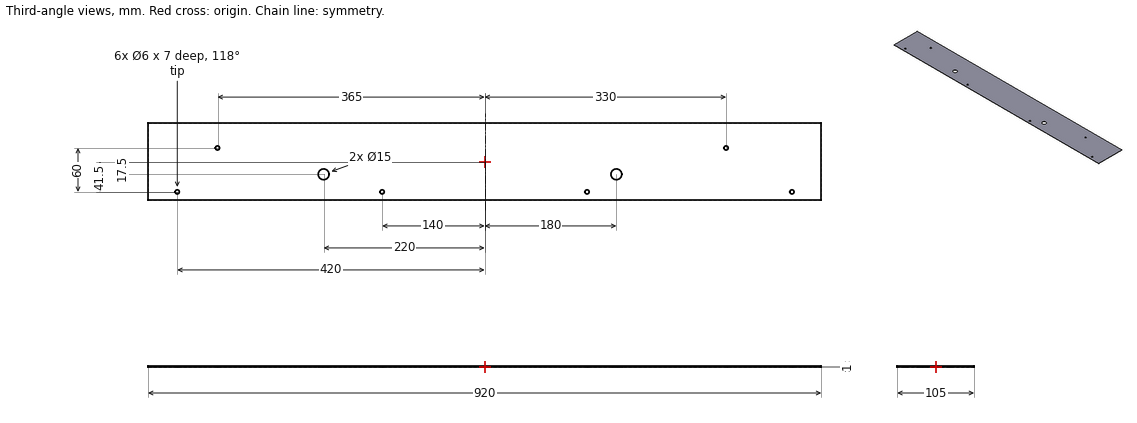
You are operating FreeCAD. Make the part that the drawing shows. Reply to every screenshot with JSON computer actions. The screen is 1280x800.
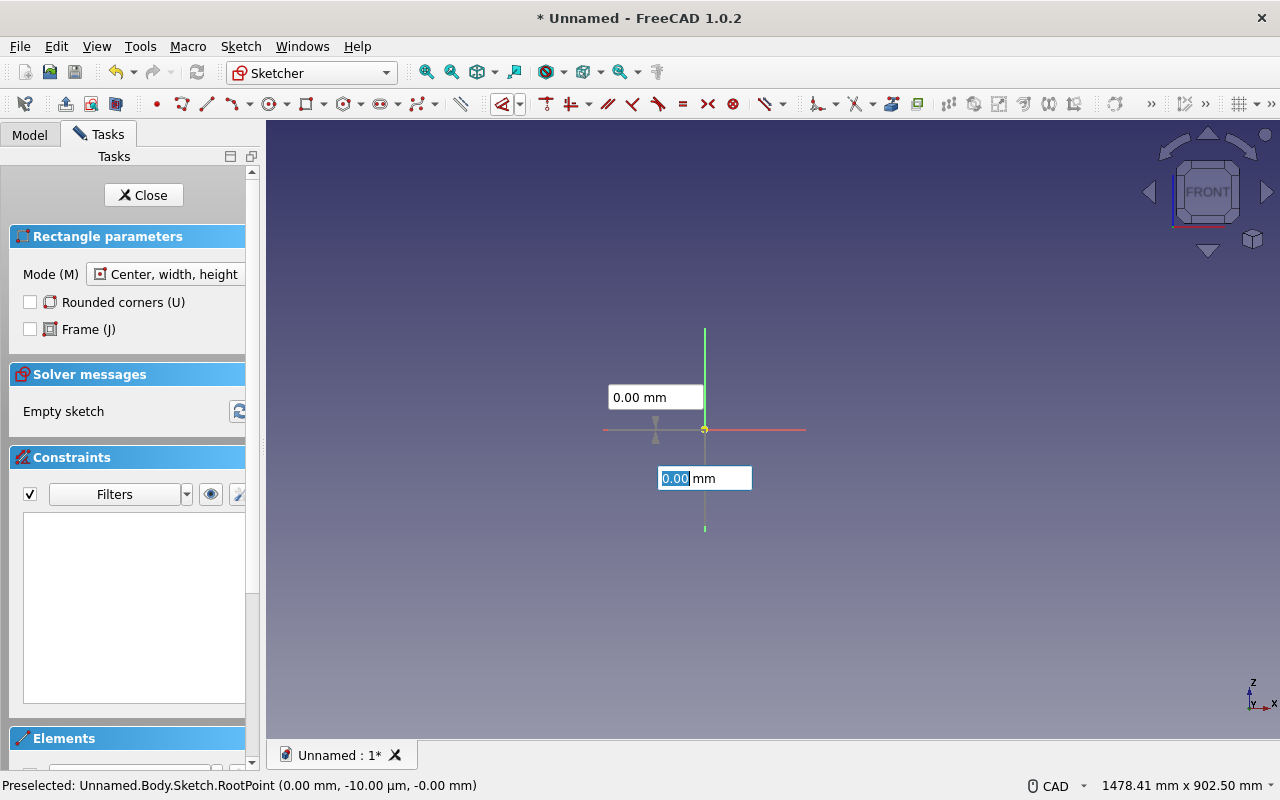
{"action": "scroll", "coordinate": [1020, 429], "scroll_direction": "up", "scroll_amount": 20}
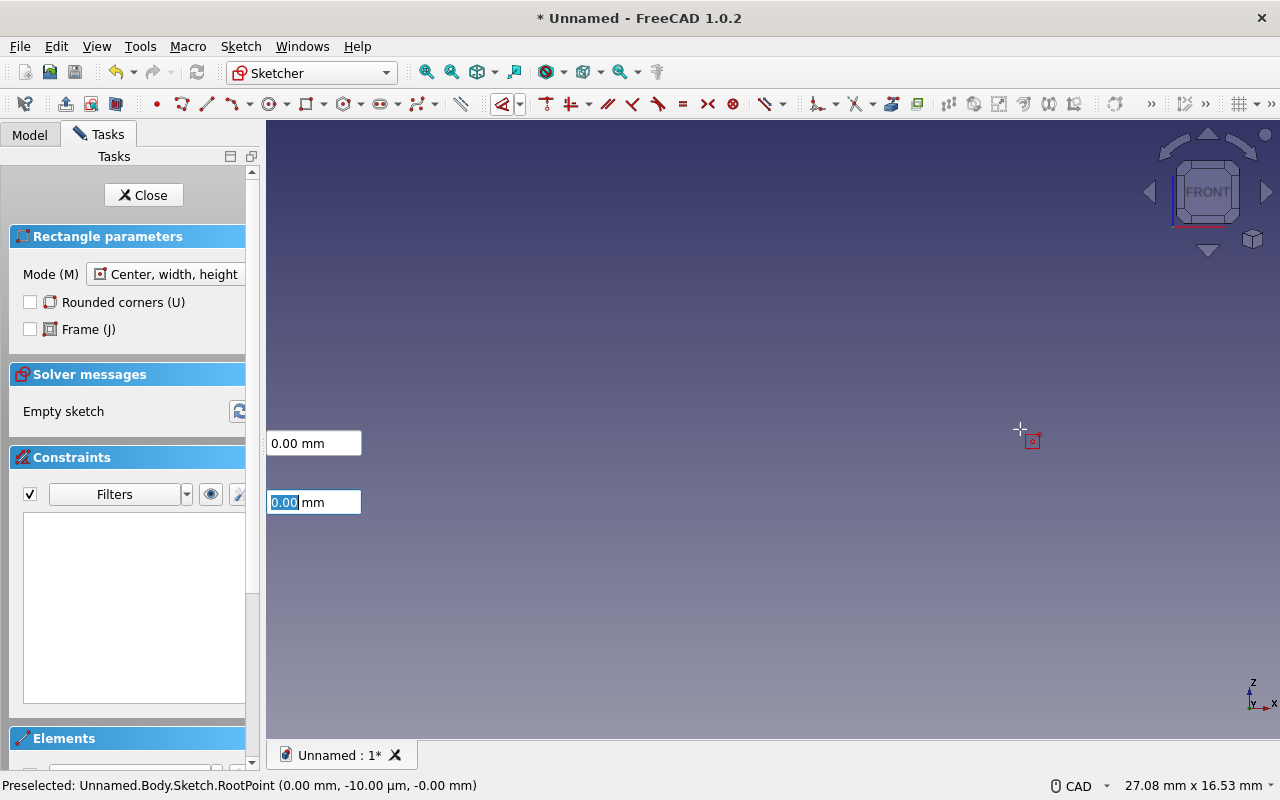
{"action": "left_click", "coordinate": [983, 425]}
{"action": "key", "text": "Escape"}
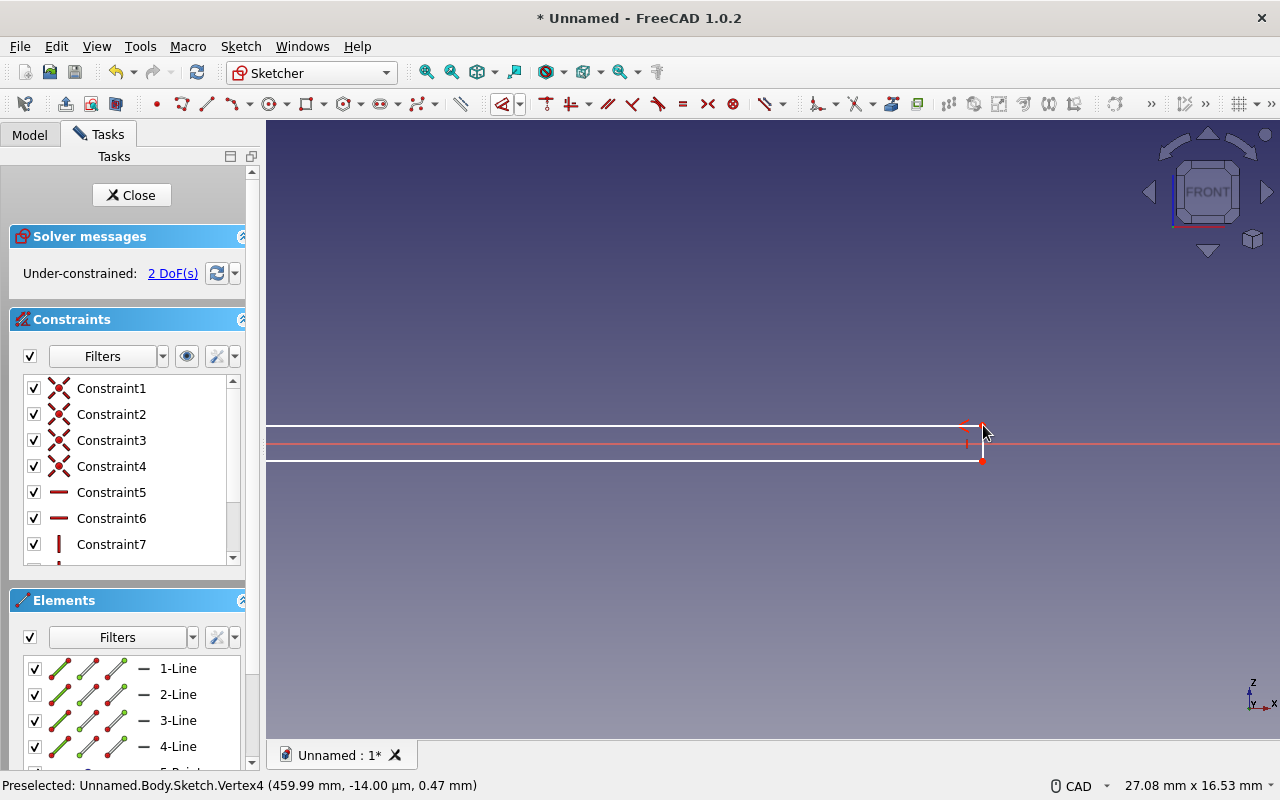
{"action": "left_click", "coordinate": [983, 447]}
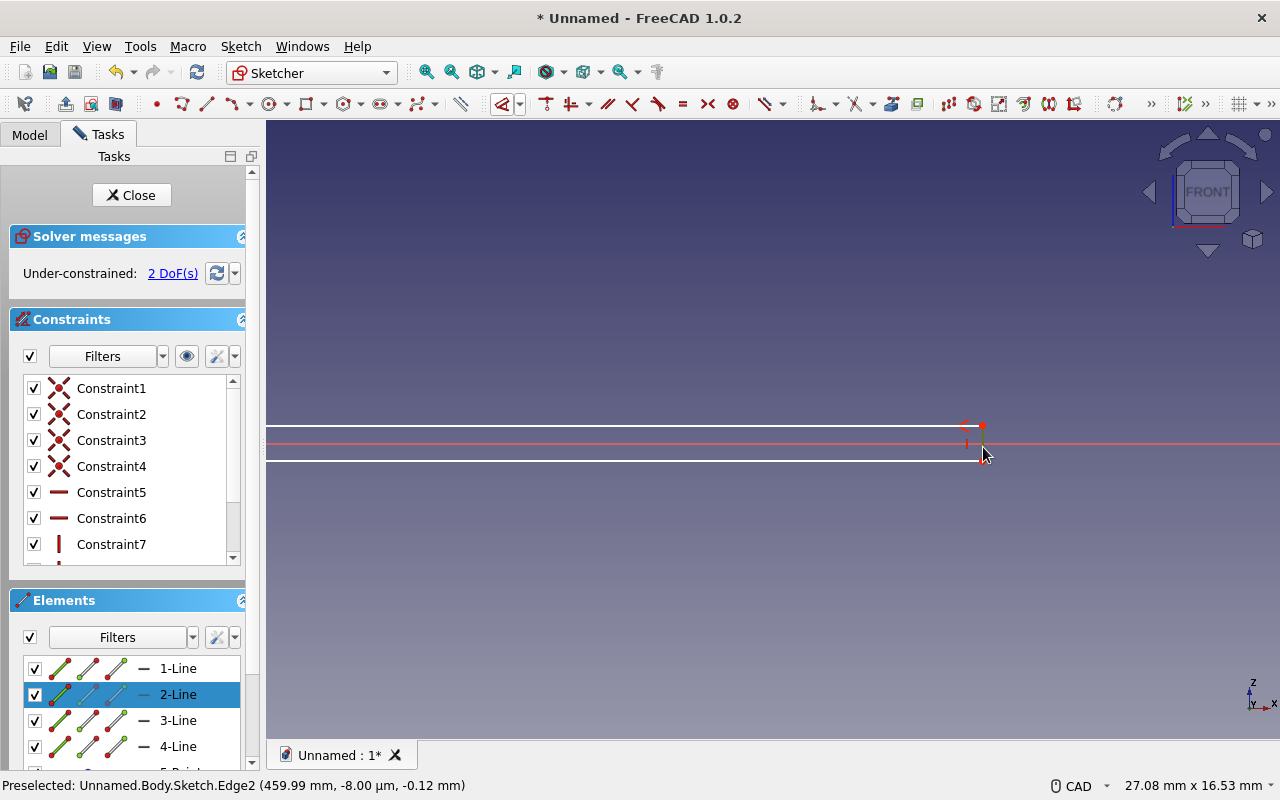
{"action": "key", "text": "i"}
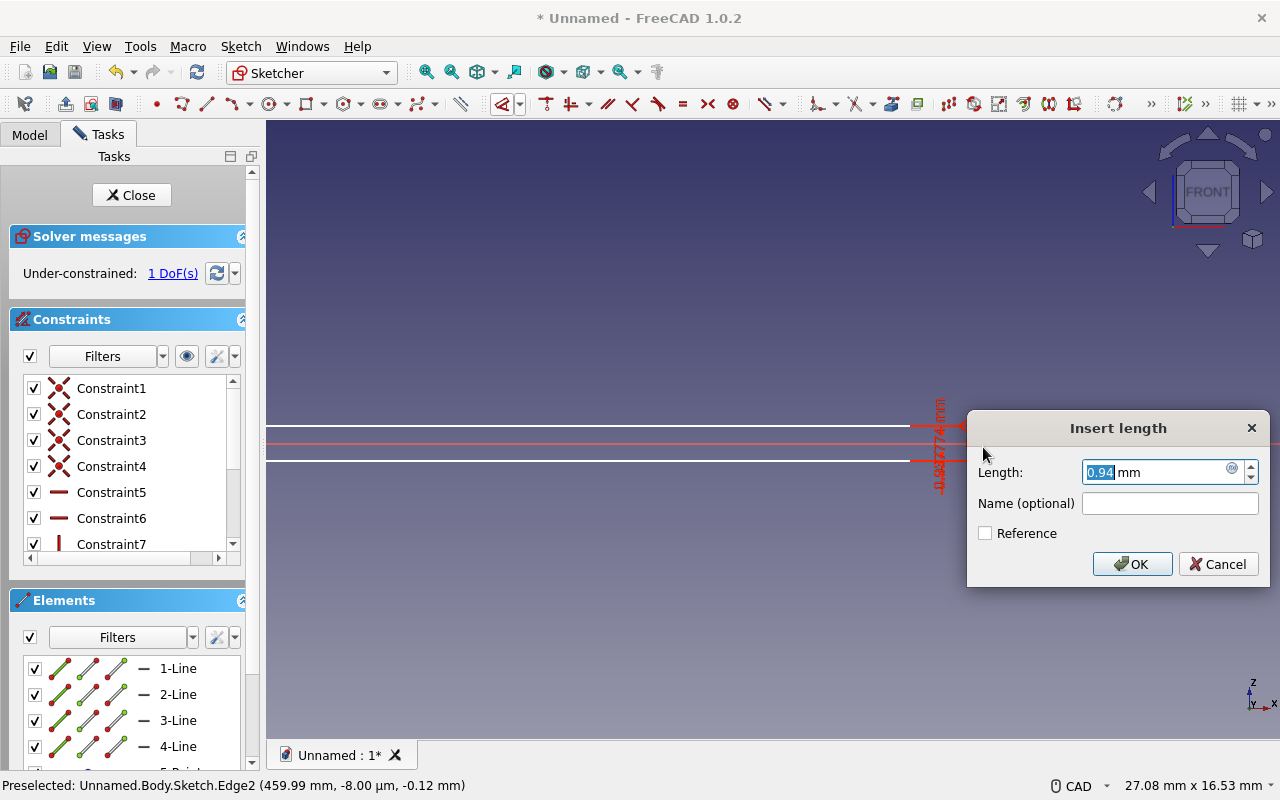
{"action": "type", "text": "1"}
{"action": "key", "text": "Return"}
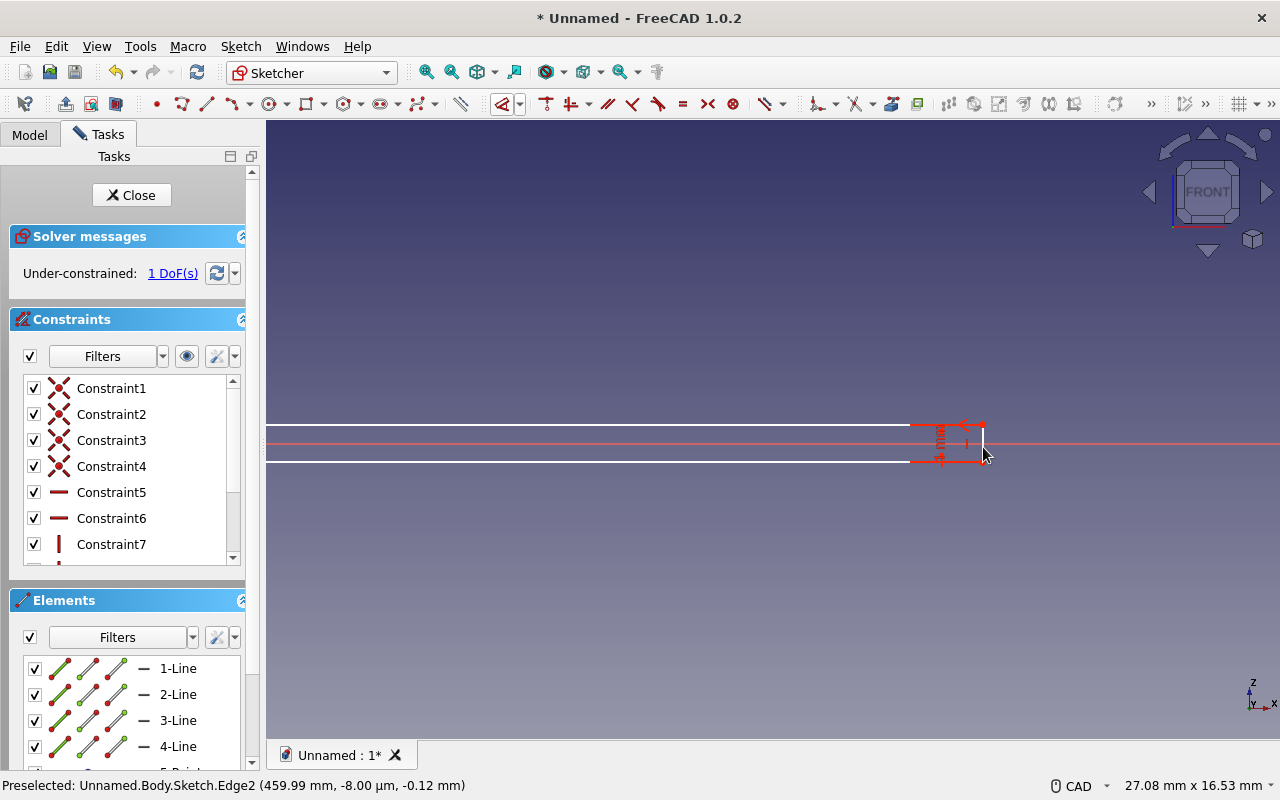
{"action": "scroll", "coordinate": [704, 430], "scroll_direction": "down", "scroll_amount": 15}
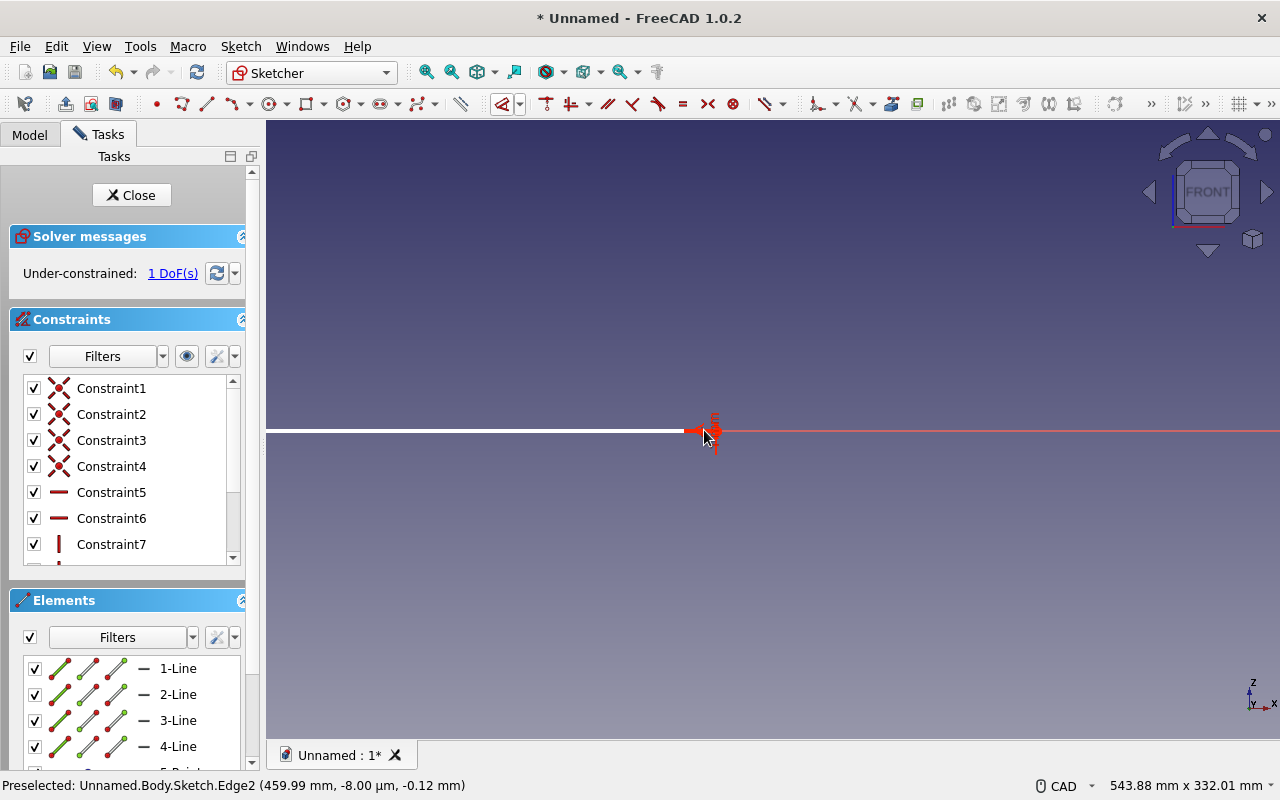
{"action": "scroll", "coordinate": [1115, 429], "scroll_direction": "down", "scroll_amount": 5}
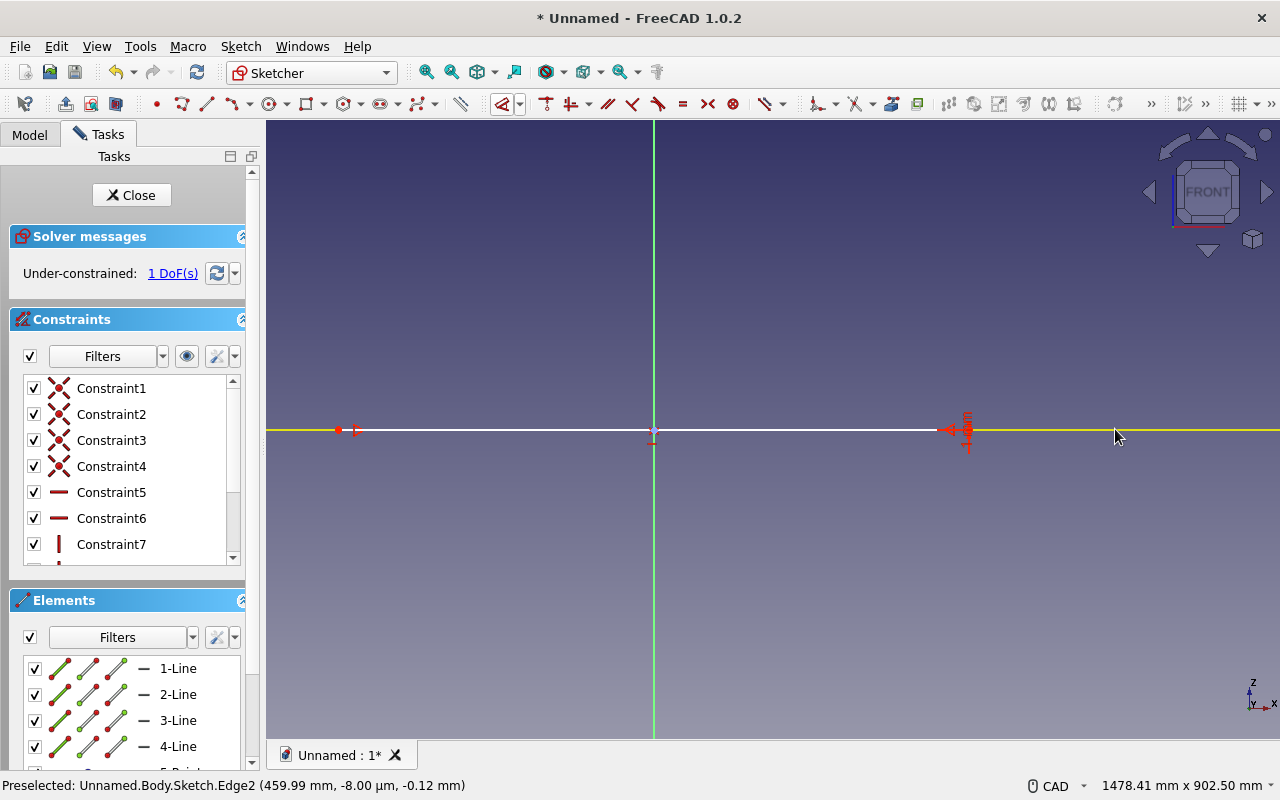
{"action": "scroll", "coordinate": [528, 430], "scroll_direction": "up", "scroll_amount": 14}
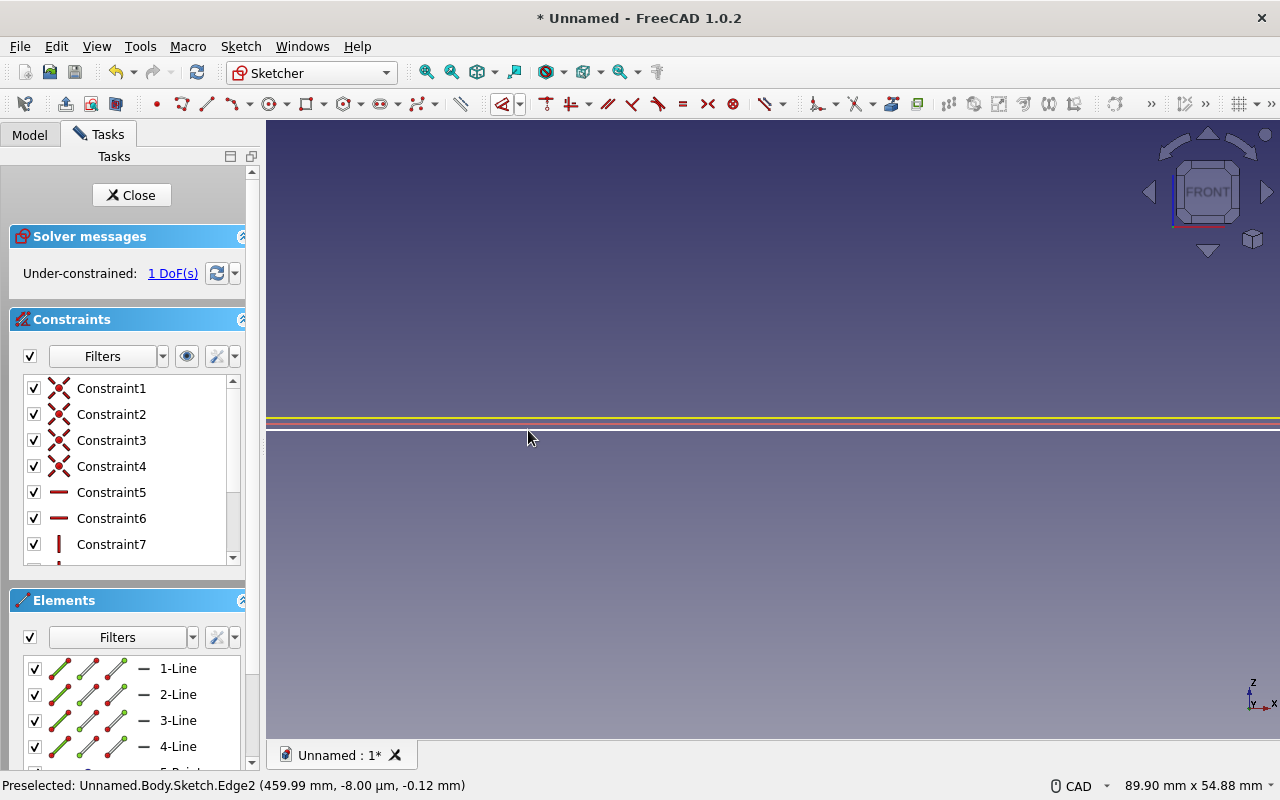
{"action": "left_click", "coordinate": [522, 430]}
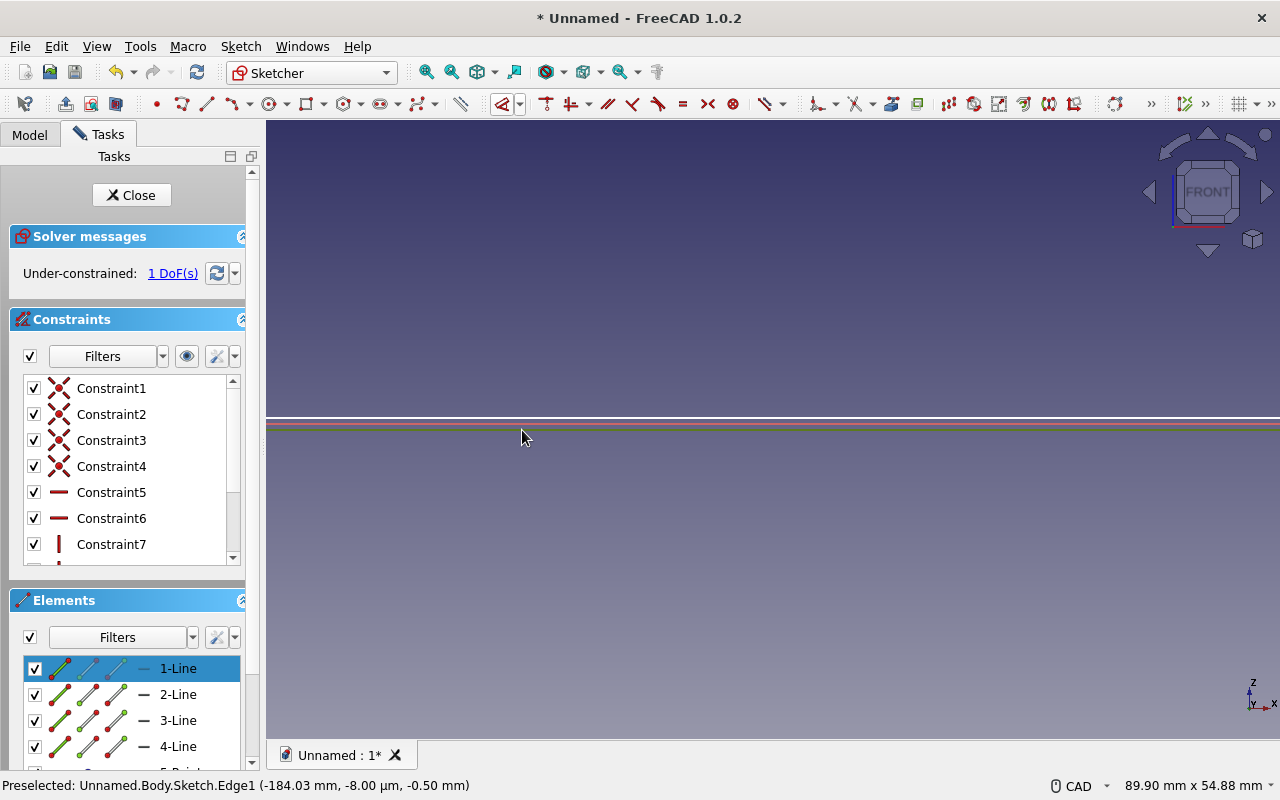
{"action": "key", "text": "l"}